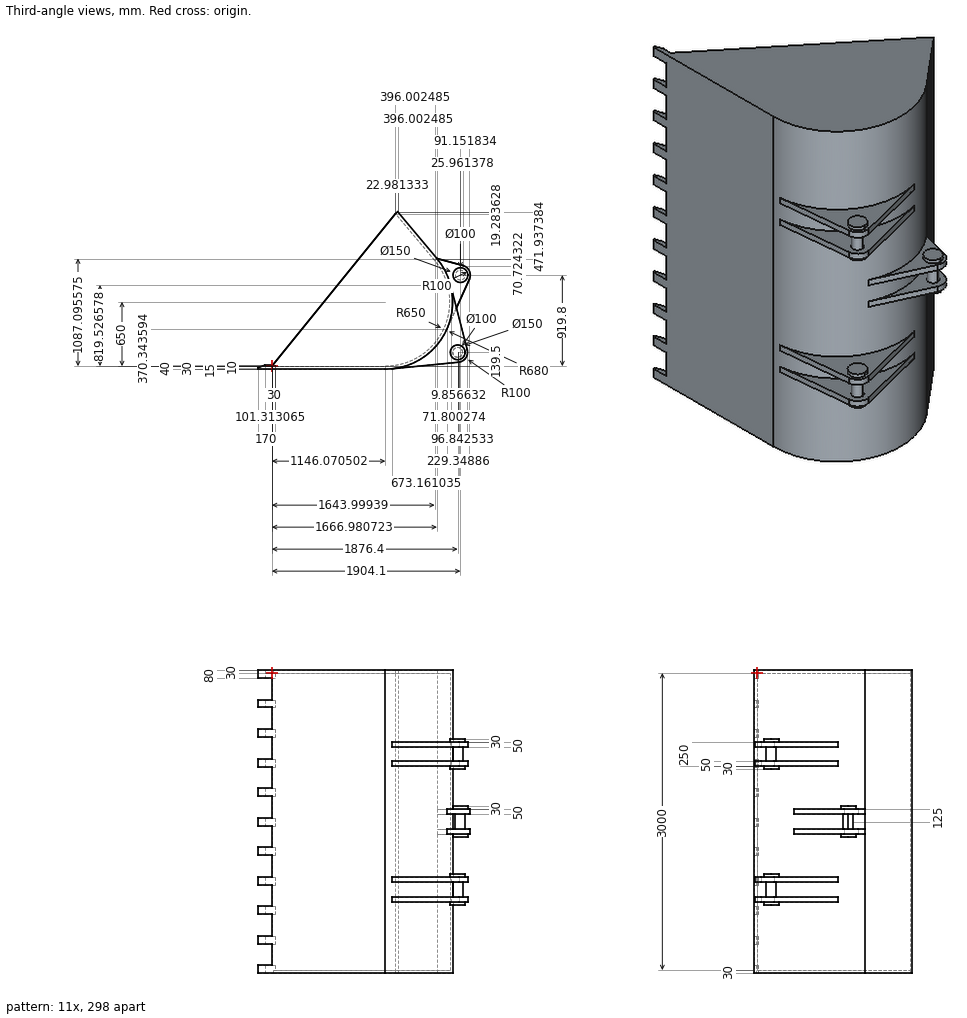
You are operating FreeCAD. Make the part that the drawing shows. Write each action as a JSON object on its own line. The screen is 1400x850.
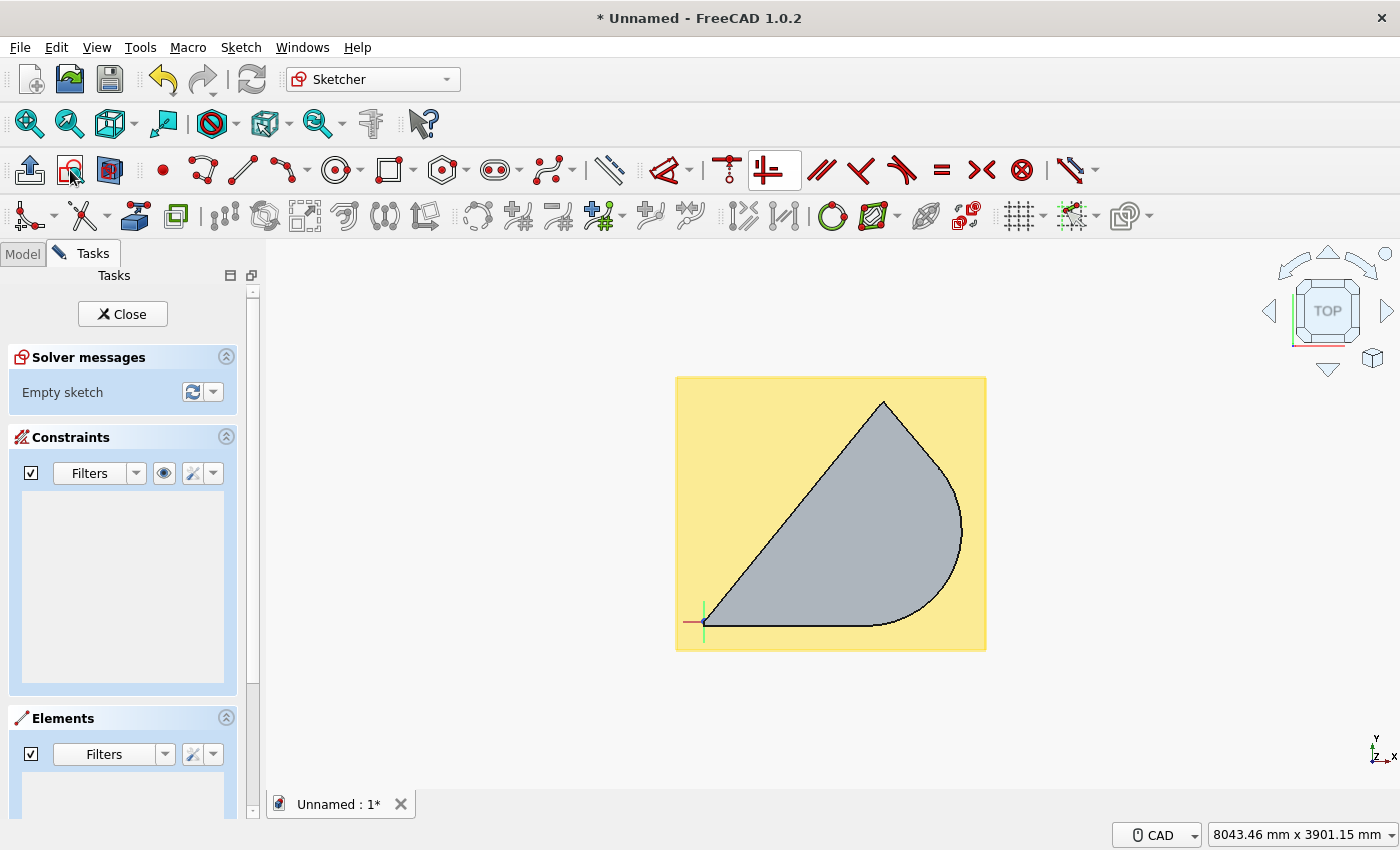
{"action": "key", "text": "q s"}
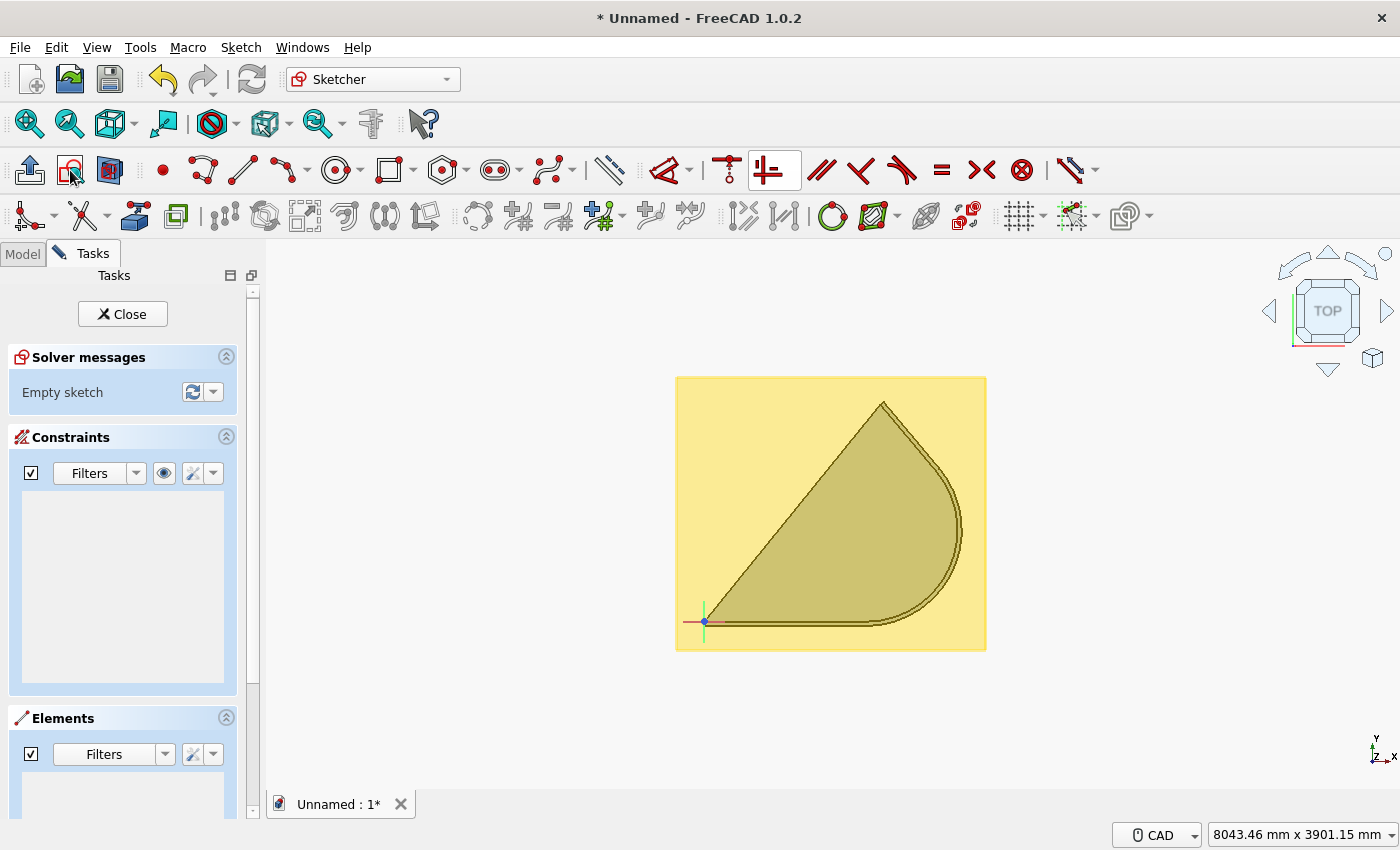
{"action": "scroll", "coordinate": [908, 608], "scroll_direction": "up", "scroll_amount": 4}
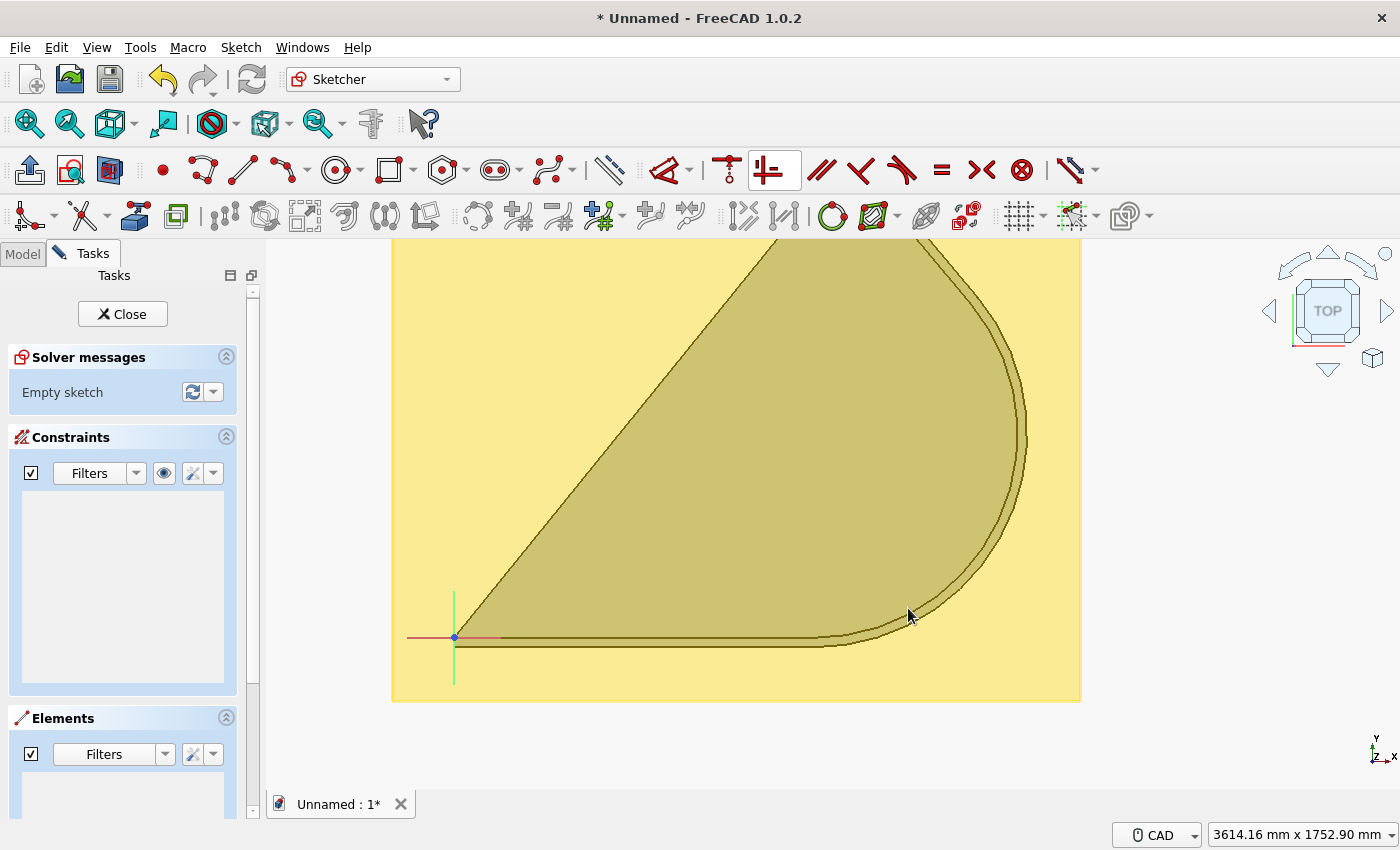
{"action": "left_click", "coordinate": [244, 170]}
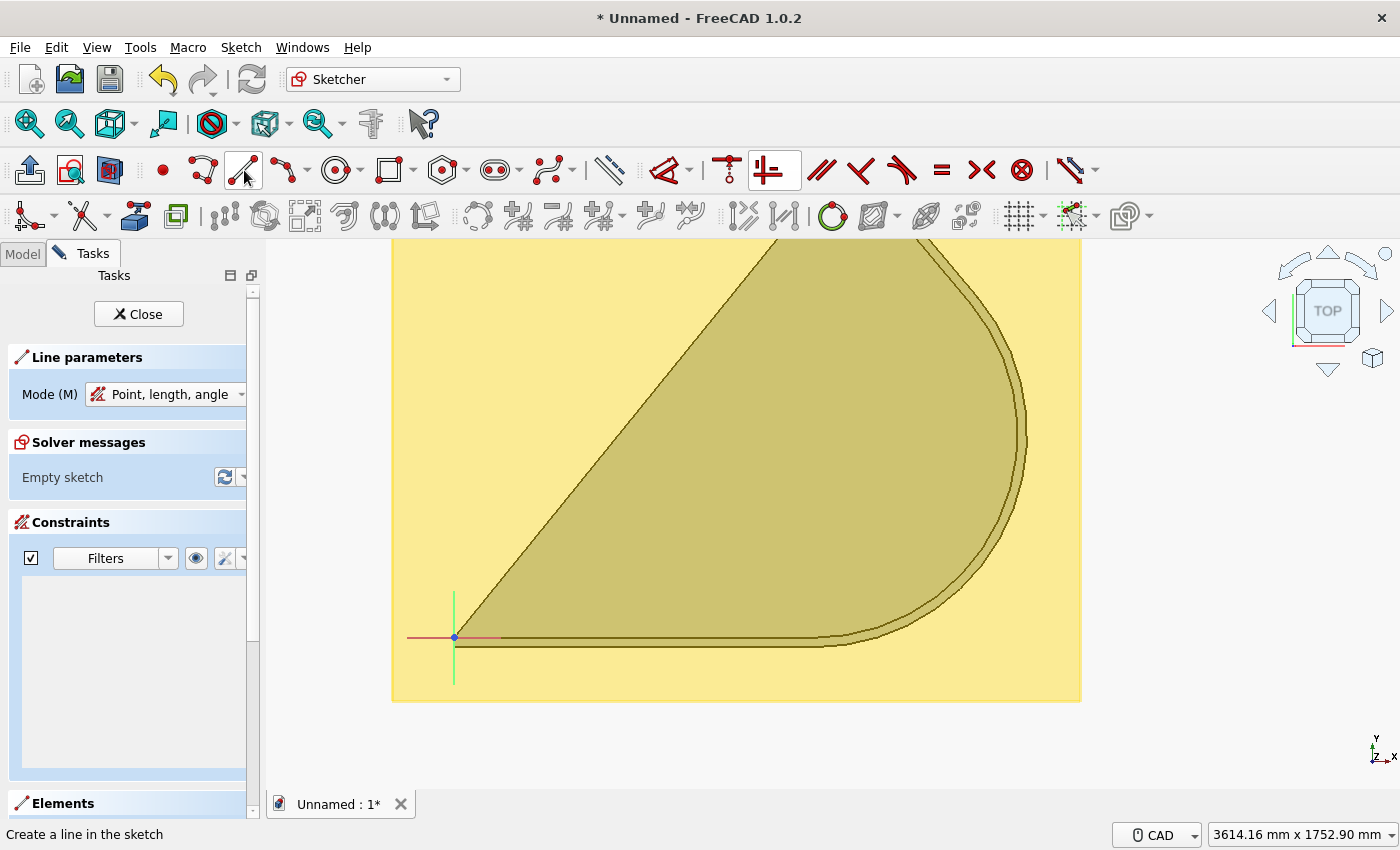
{"action": "scroll", "coordinate": [835, 646], "scroll_direction": "up", "scroll_amount": 4}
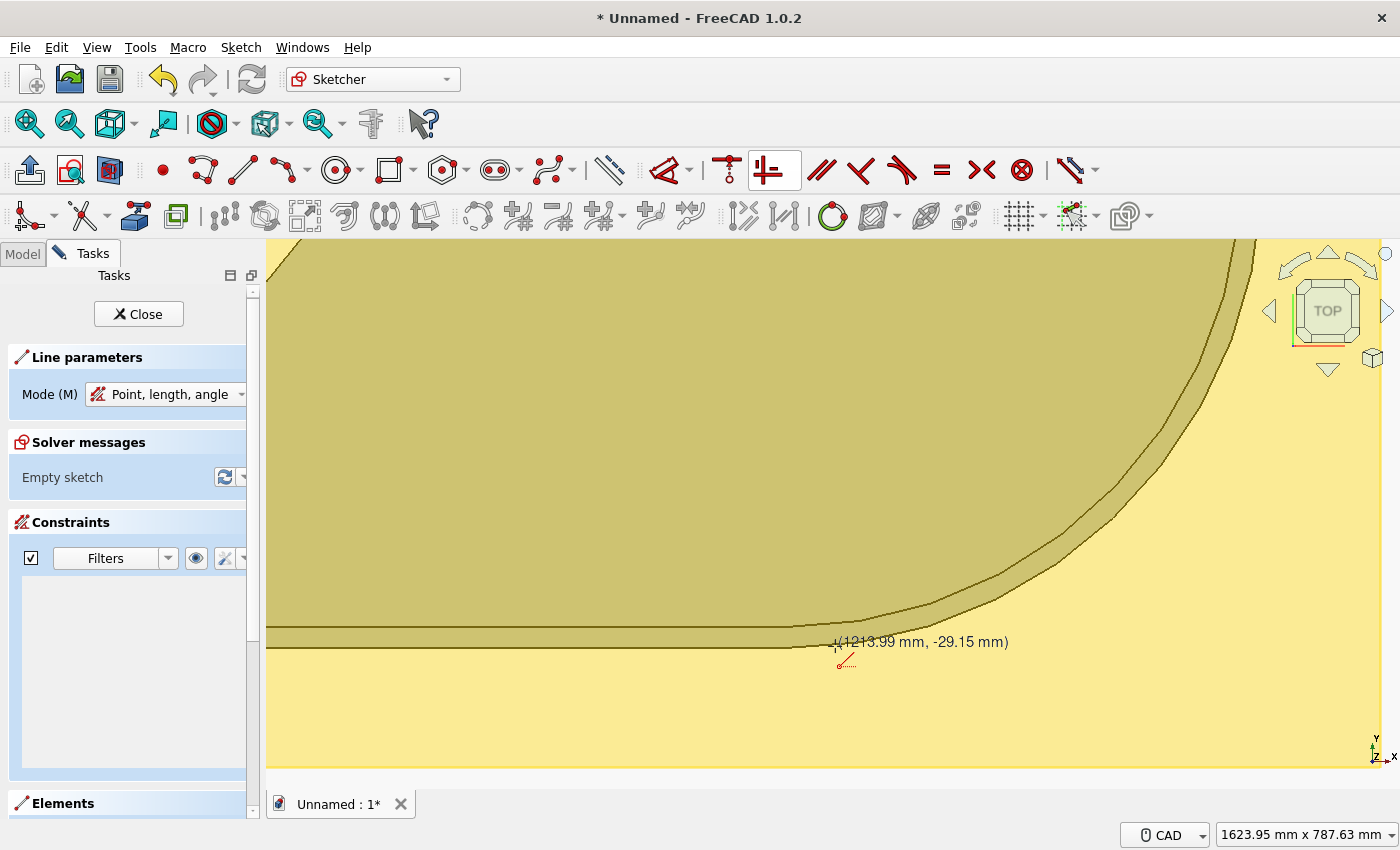
{"action": "left_click", "coordinate": [834, 646]}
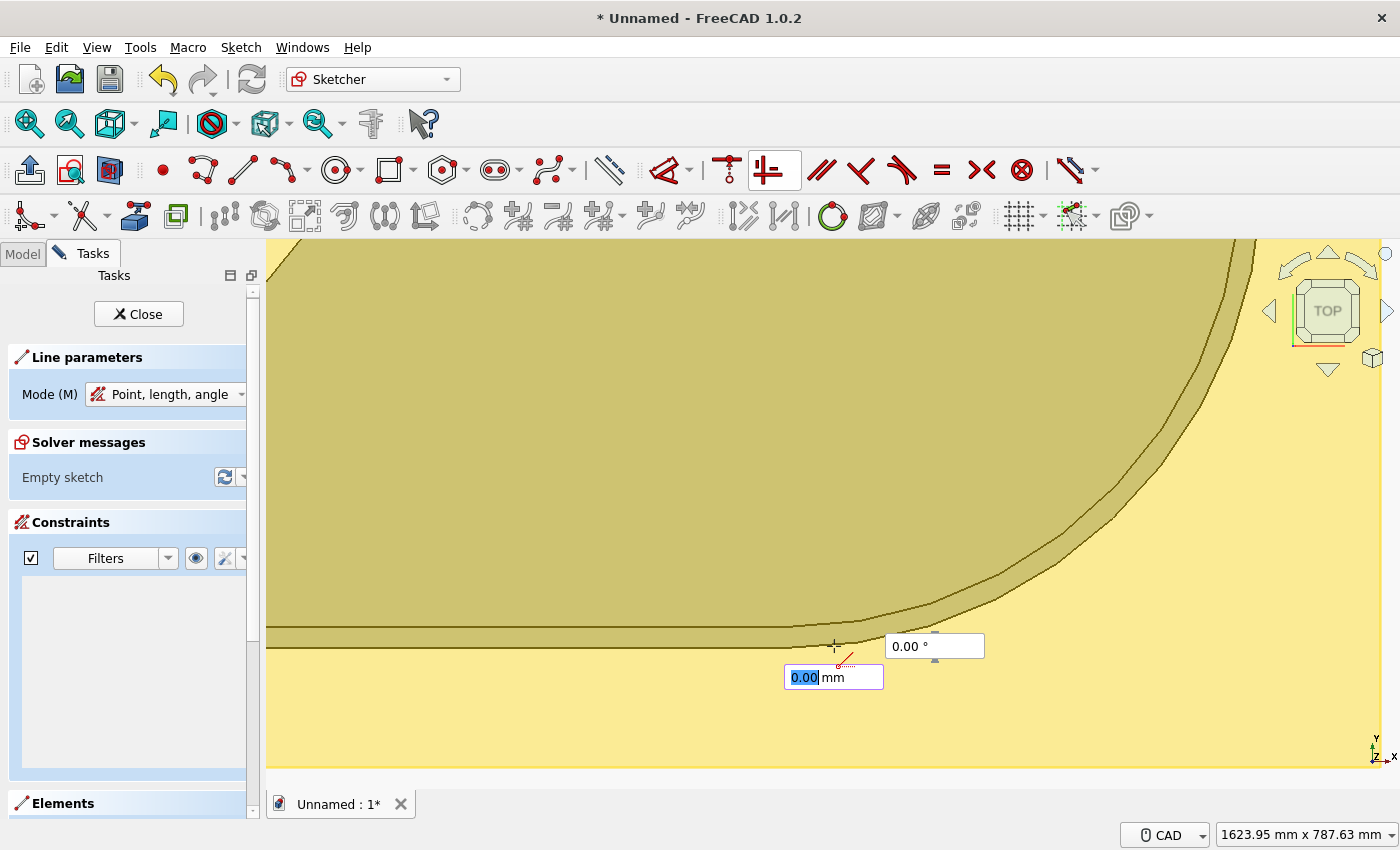
{"action": "scroll", "coordinate": [837, 648], "scroll_direction": "down", "scroll_amount": 4}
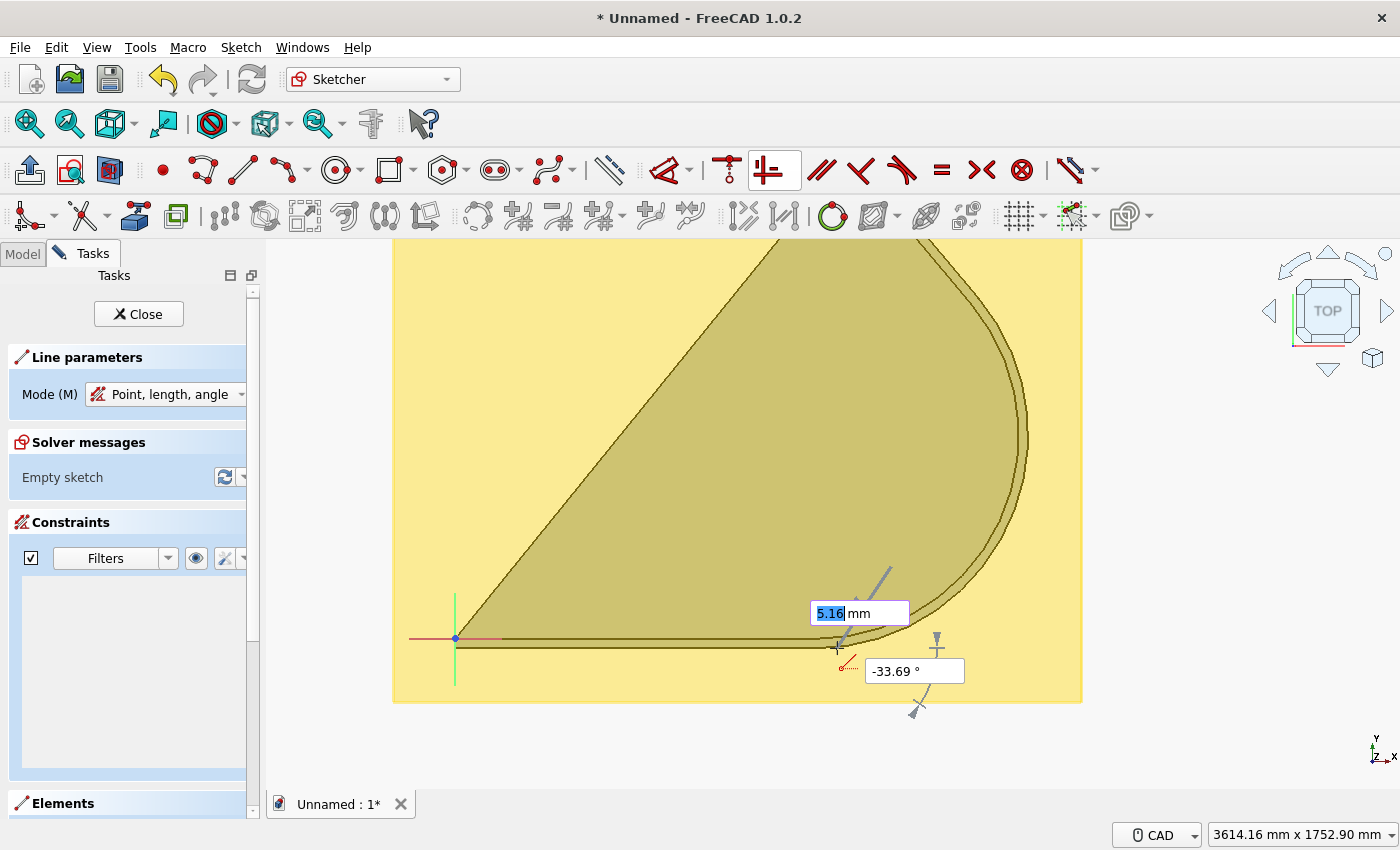
{"action": "scroll", "coordinate": [1047, 626], "scroll_direction": "up", "scroll_amount": 2}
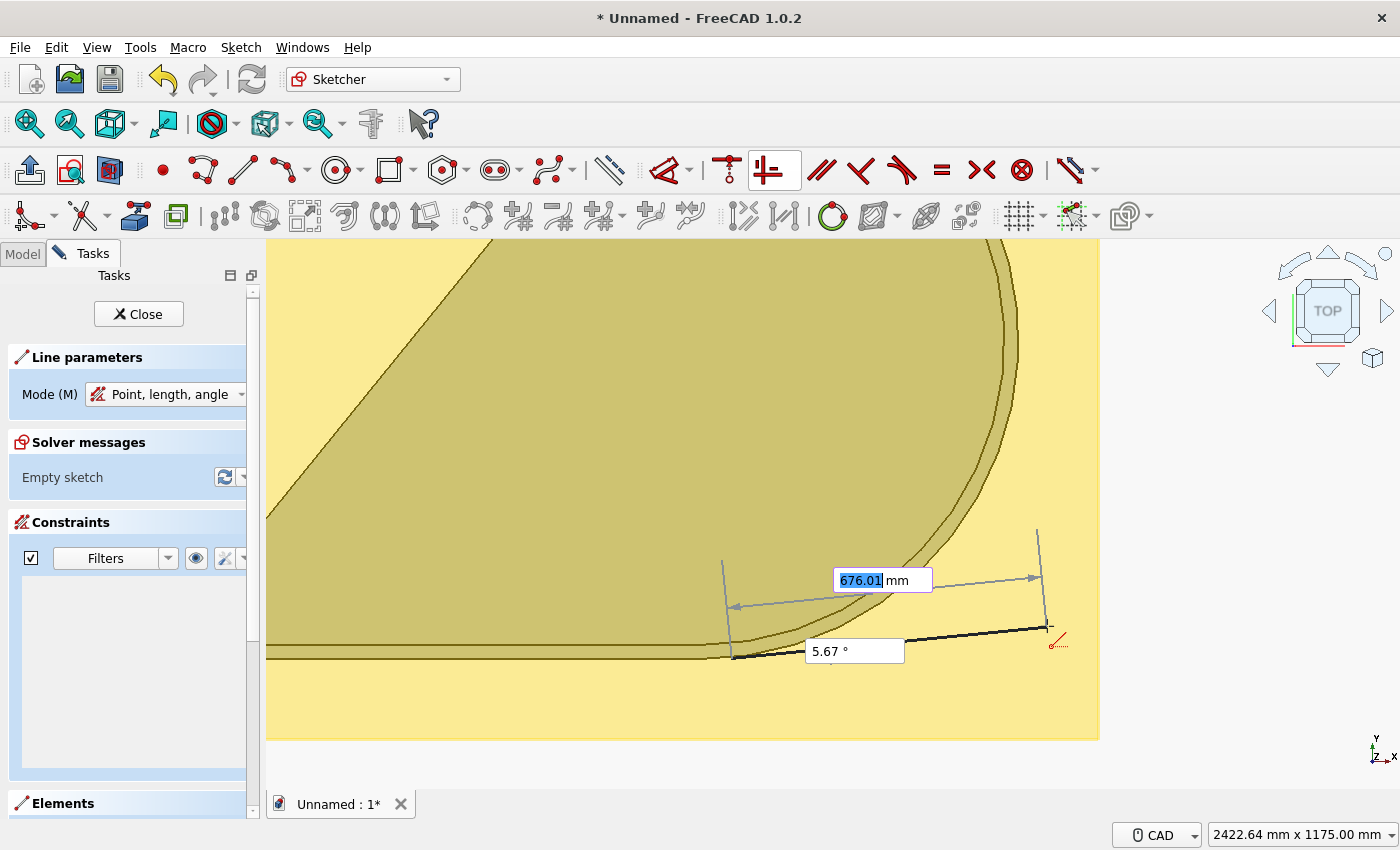
{"action": "left_click", "coordinate": [1047, 626]}